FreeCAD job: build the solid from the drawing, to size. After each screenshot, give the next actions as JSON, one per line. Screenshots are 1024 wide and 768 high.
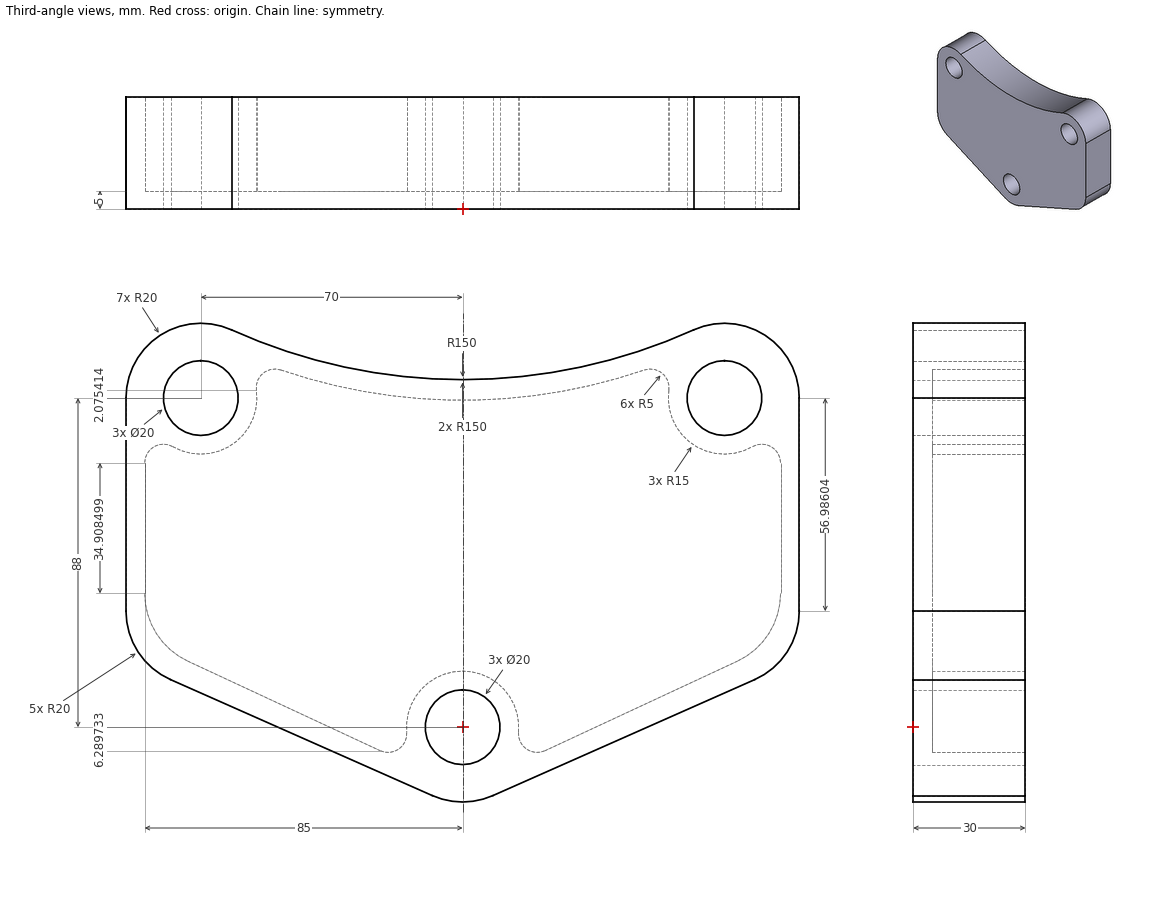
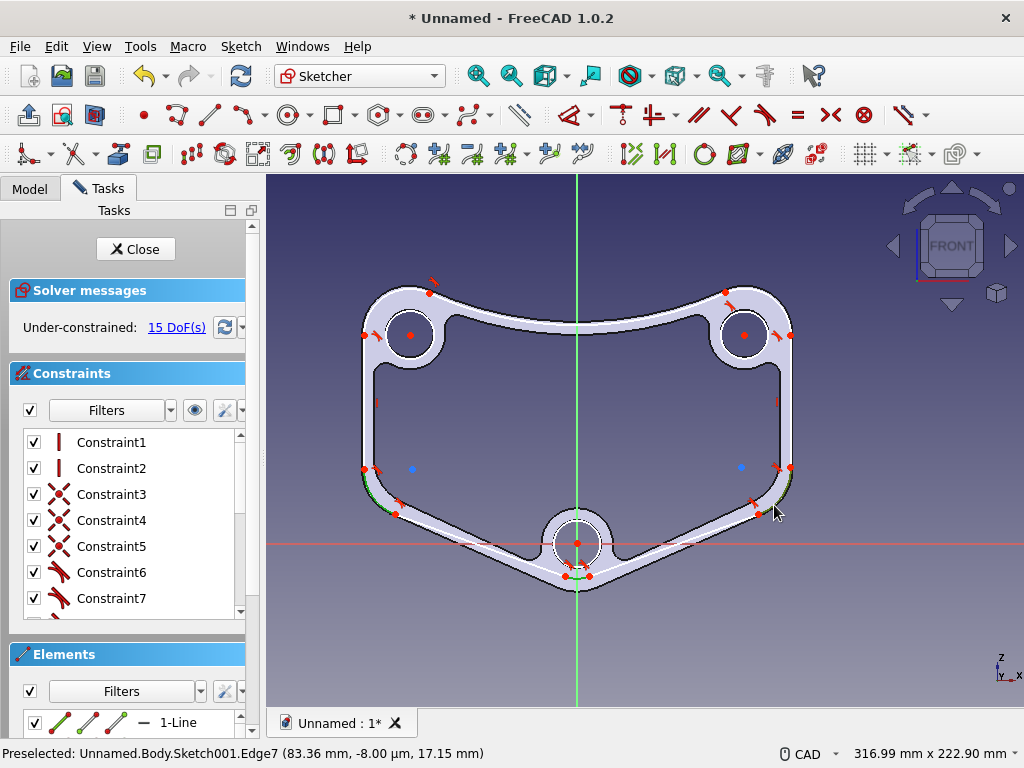
{"action": "left_click", "coordinate": [783, 309]}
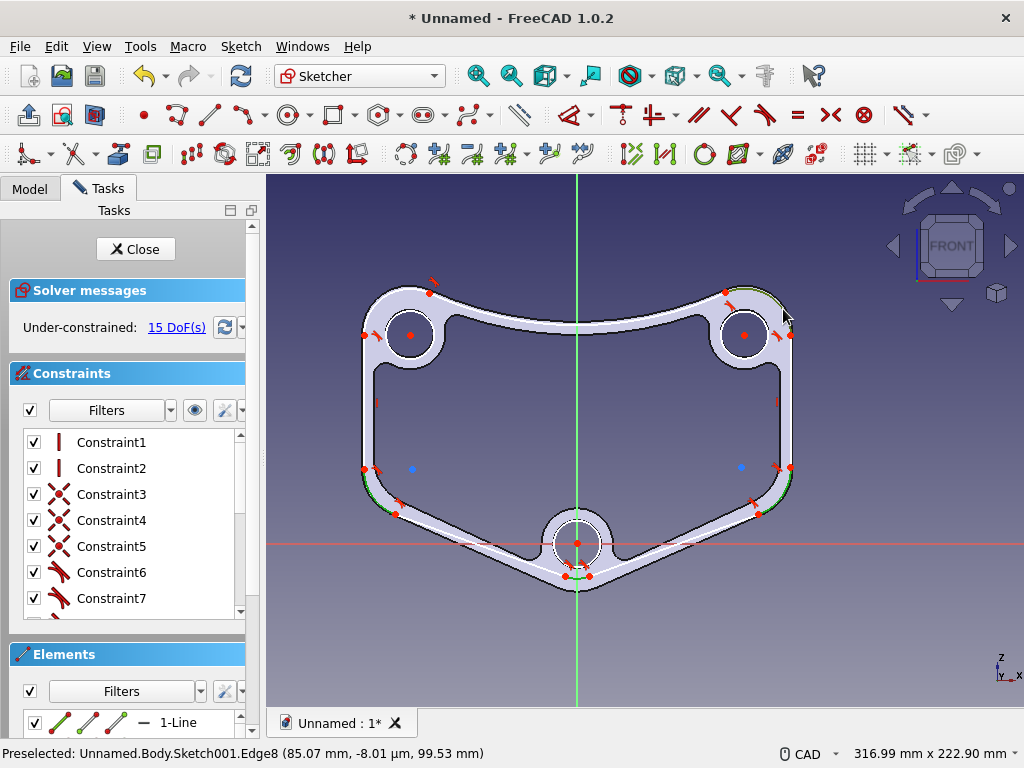
{"action": "left_click", "coordinate": [402, 290]}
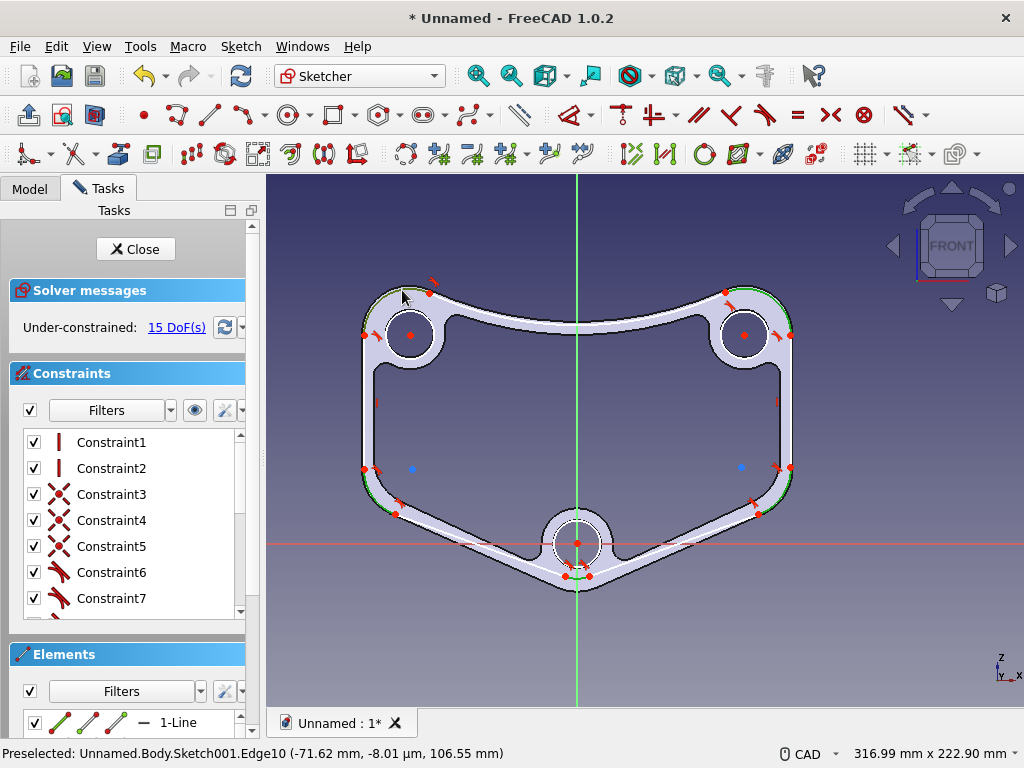
{"action": "left_click", "coordinate": [798, 116]}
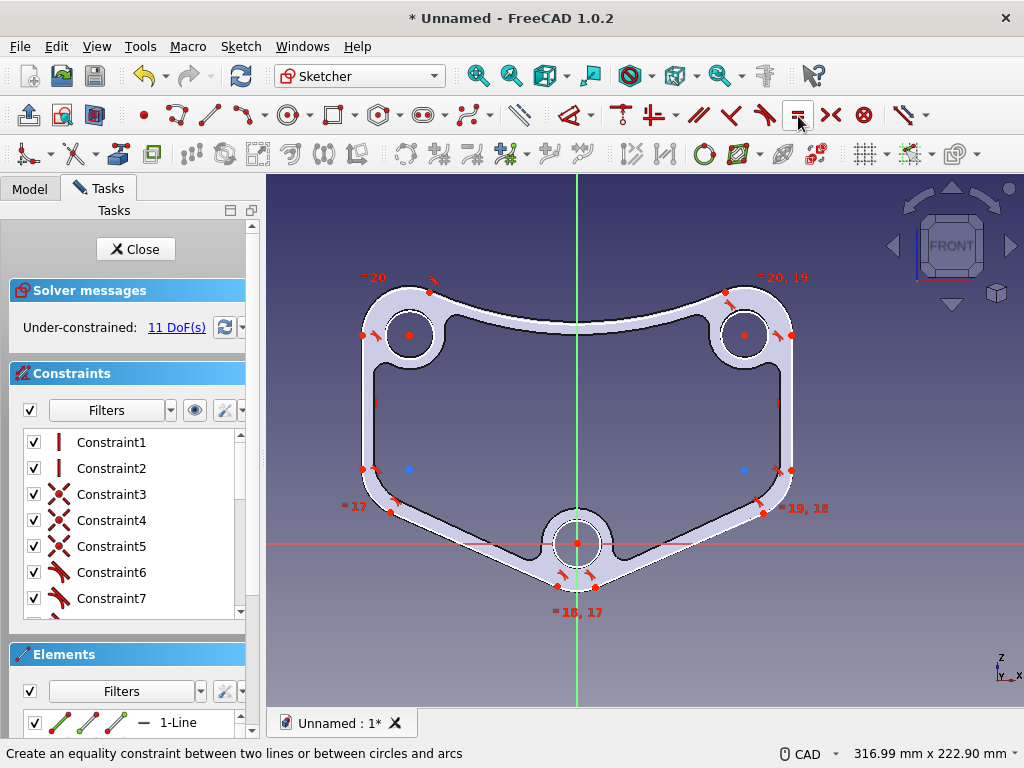
{"action": "left_click", "coordinate": [594, 528]}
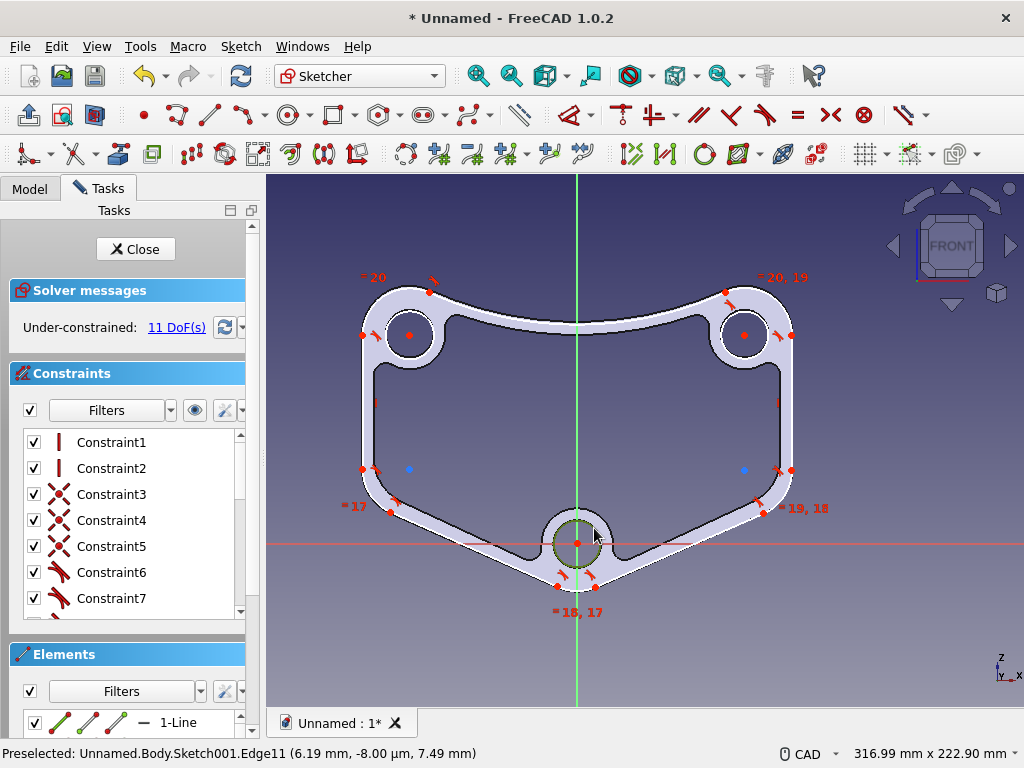
{"action": "left_click", "coordinate": [427, 318]}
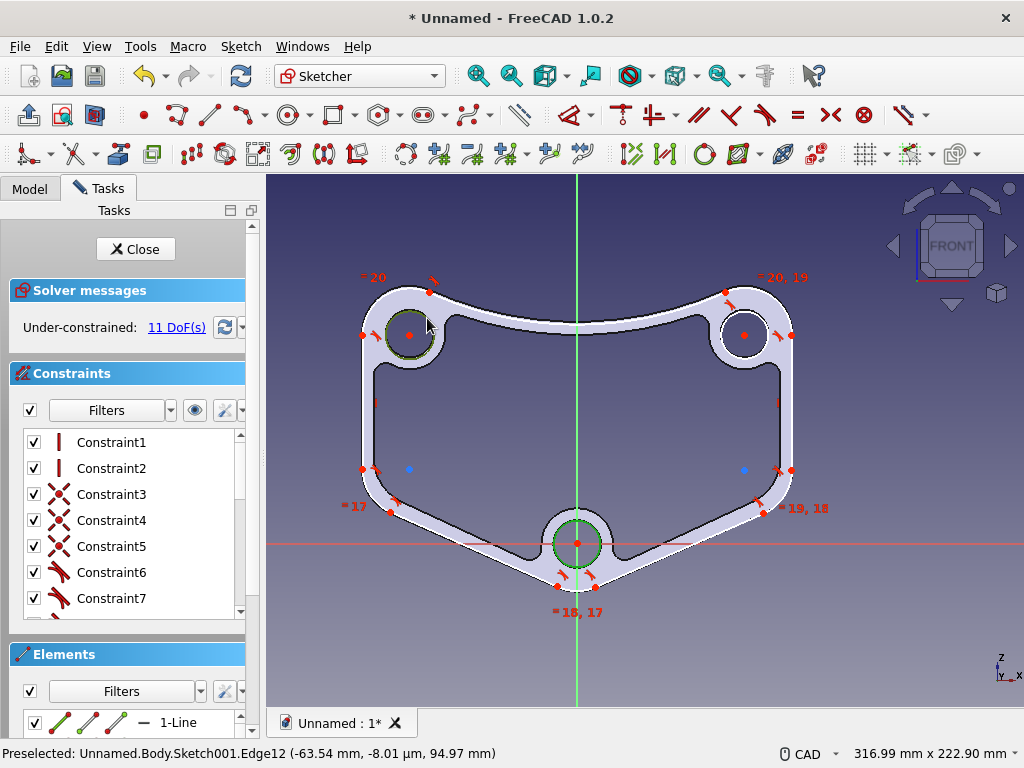
{"action": "left_click", "coordinate": [761, 318]}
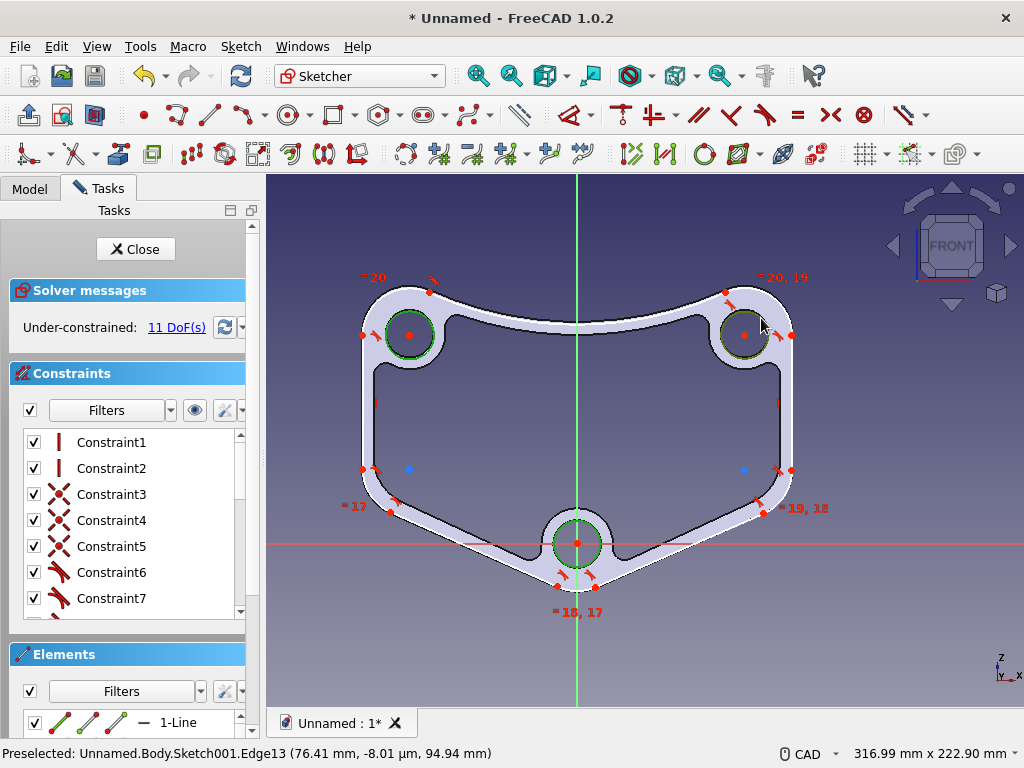
{"action": "left_click", "coordinate": [798, 116]}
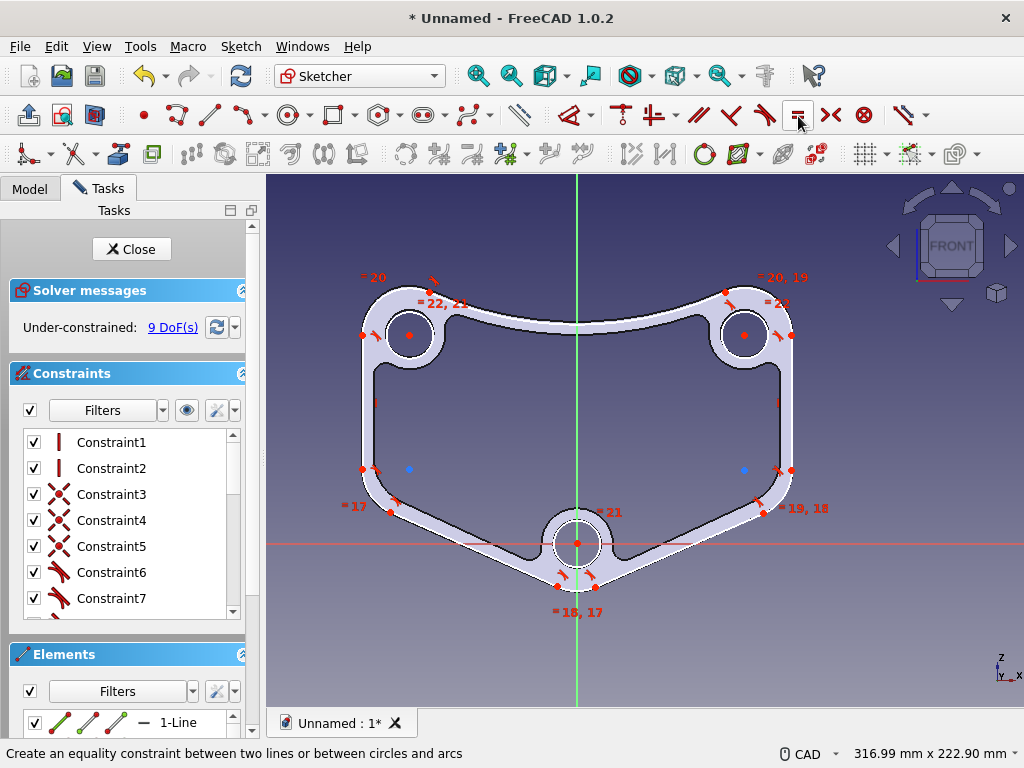
{"action": "scroll", "coordinate": [576, 636], "scroll_direction": "down", "scroll_amount": 3}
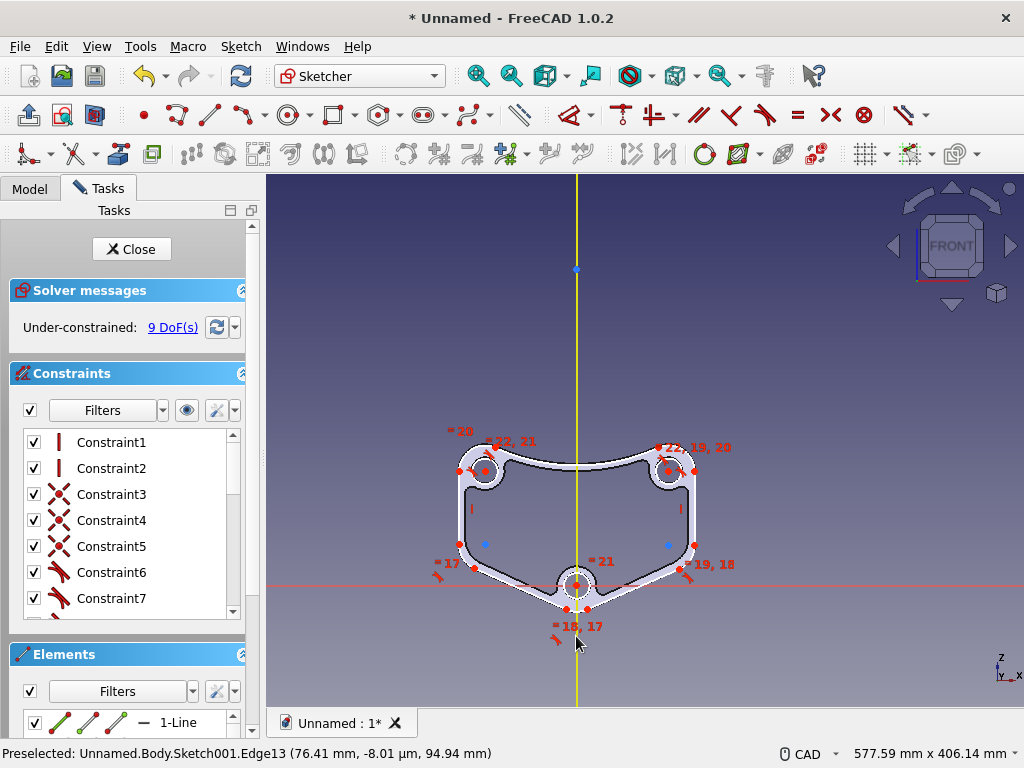
{"action": "left_click", "coordinate": [577, 270]}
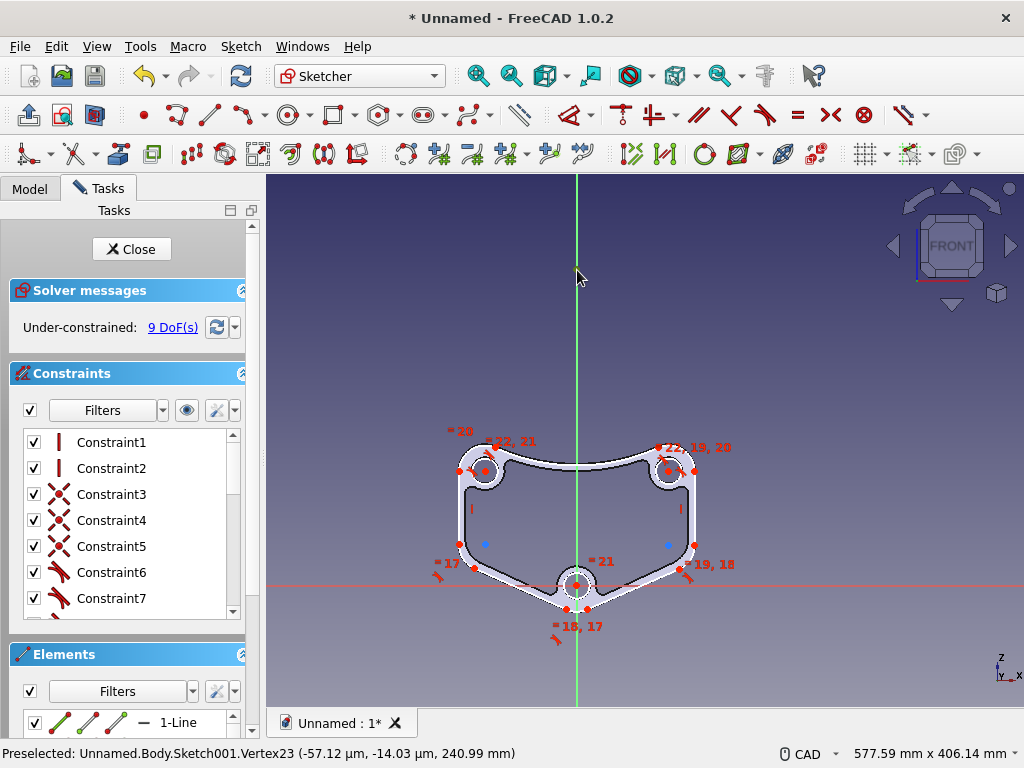
{"action": "left_click", "coordinate": [577, 543]}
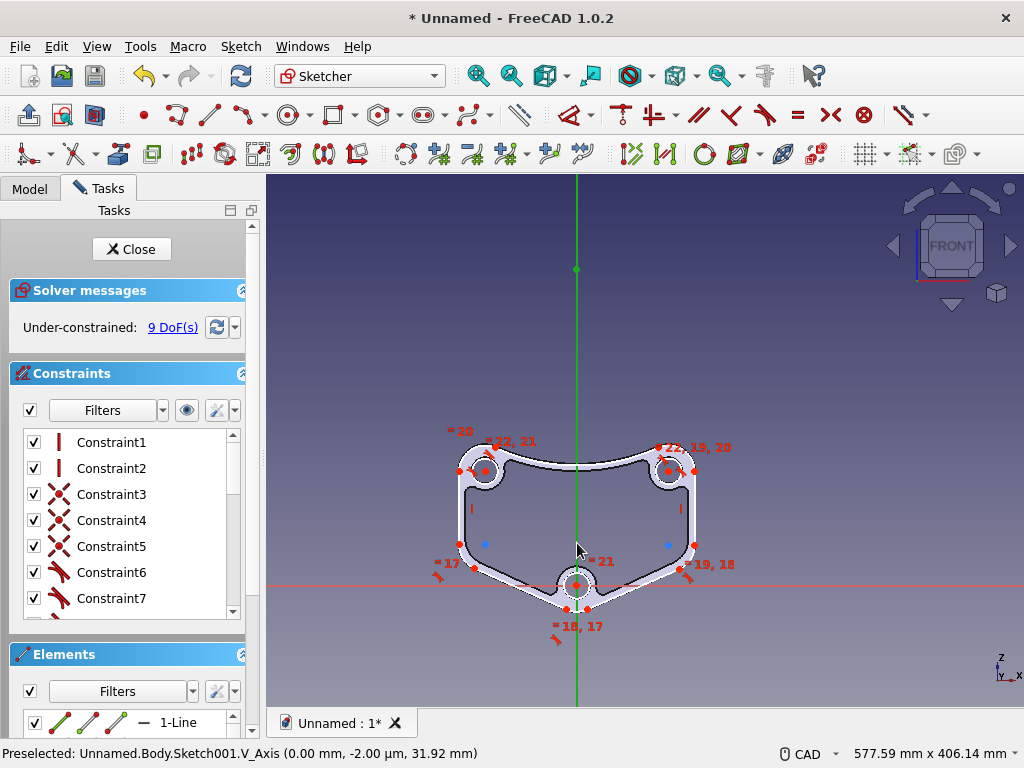
{"action": "left_click", "coordinate": [621, 116]}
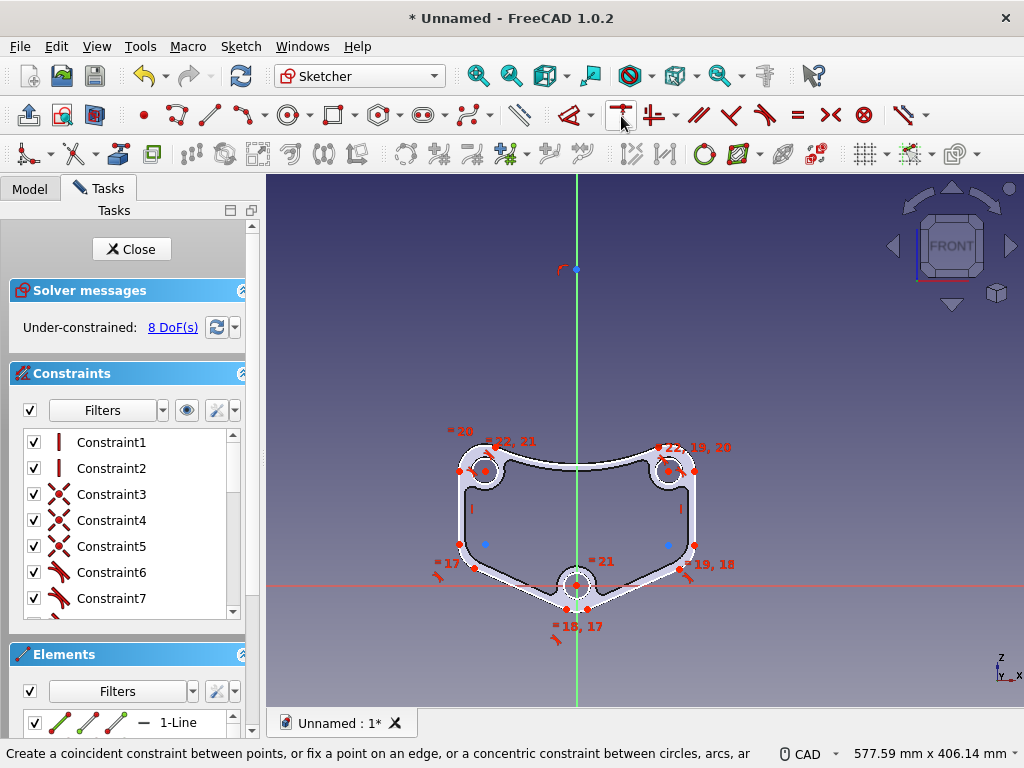
{"action": "left_click", "coordinate": [485, 545]}